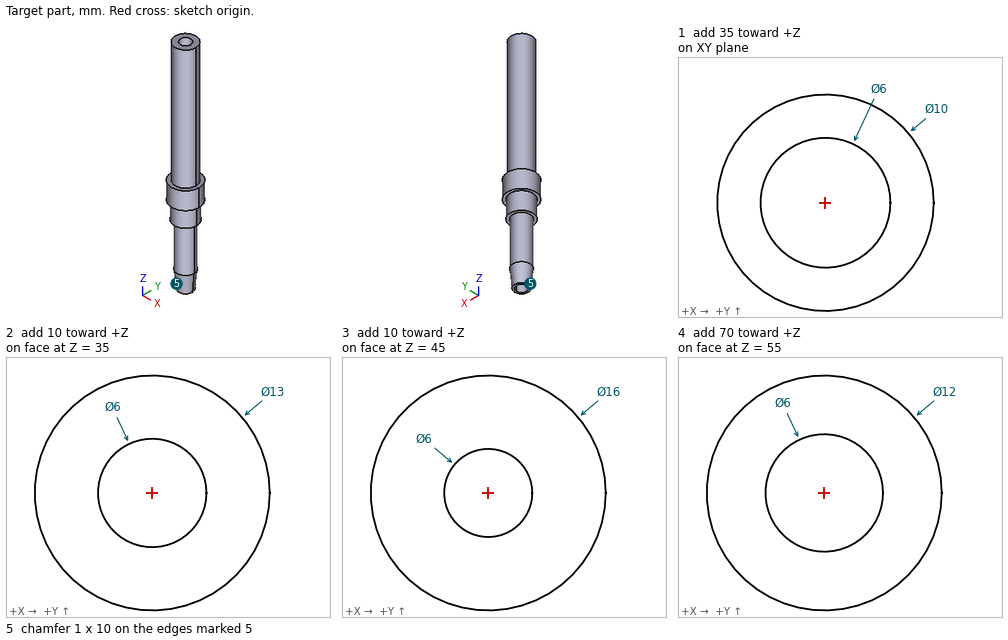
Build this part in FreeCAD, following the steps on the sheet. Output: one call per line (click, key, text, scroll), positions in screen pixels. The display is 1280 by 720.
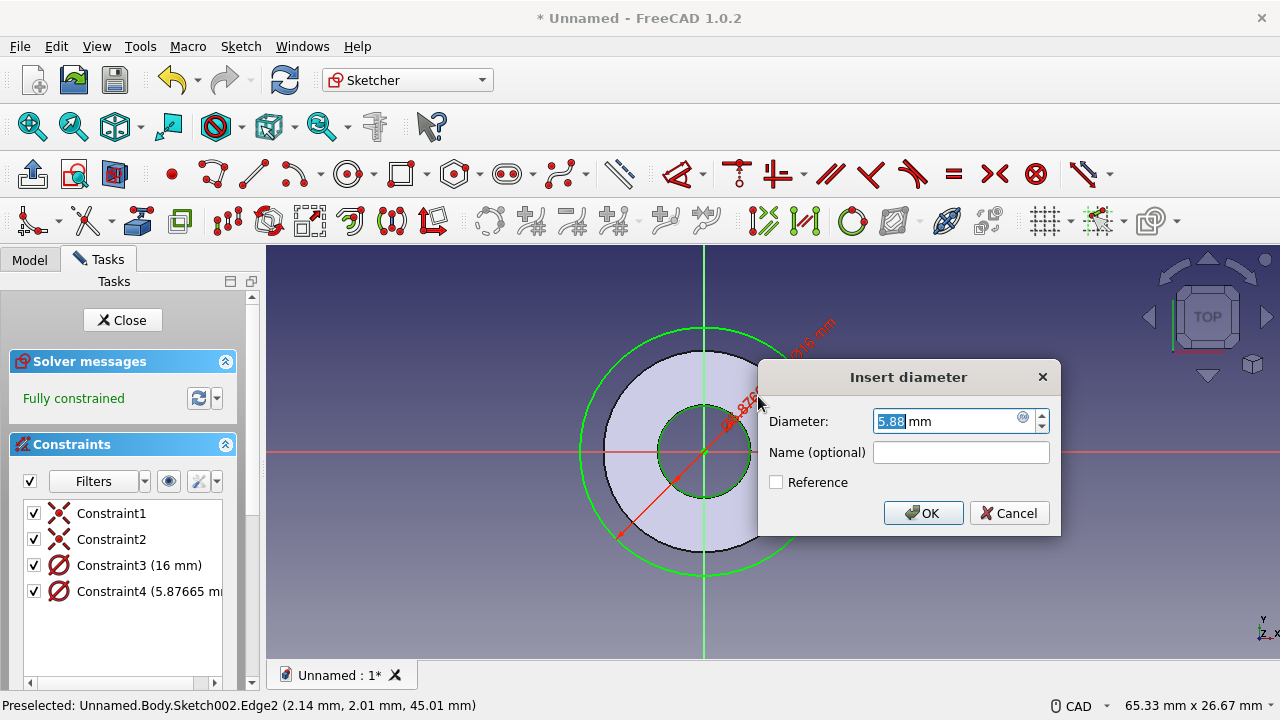
text(6)
key(Return)
key(Escape)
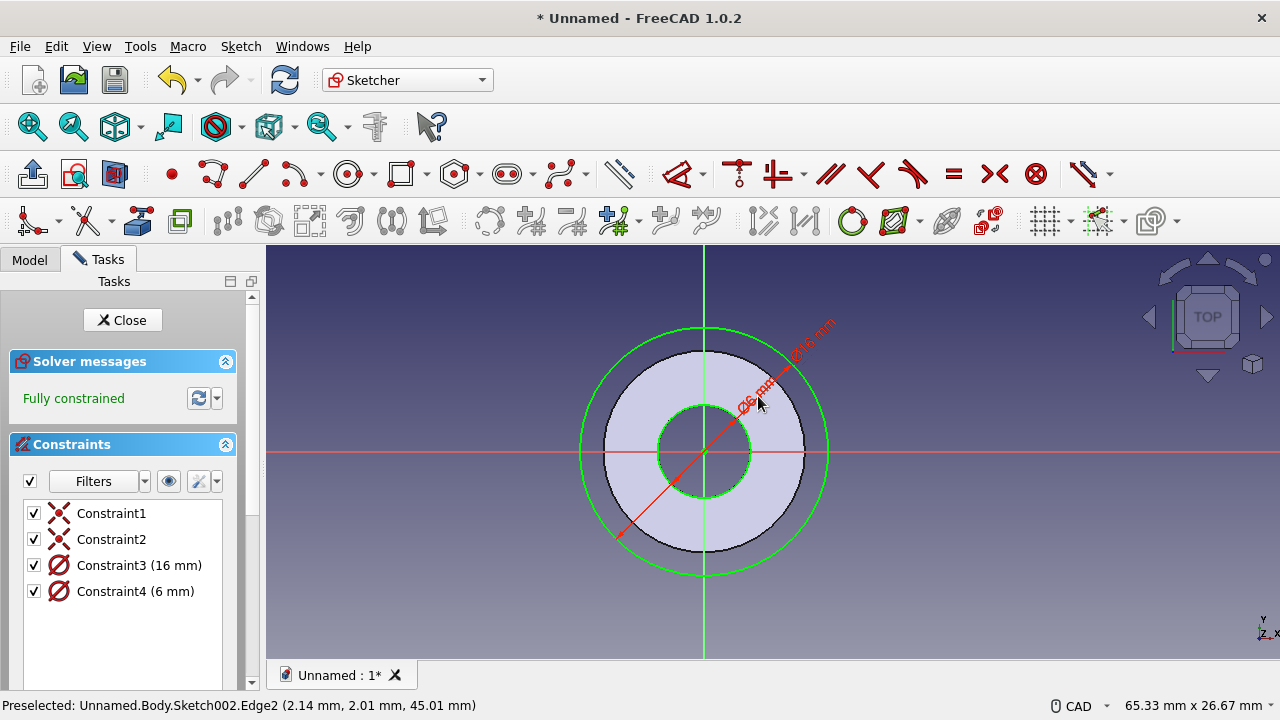
click(123, 320)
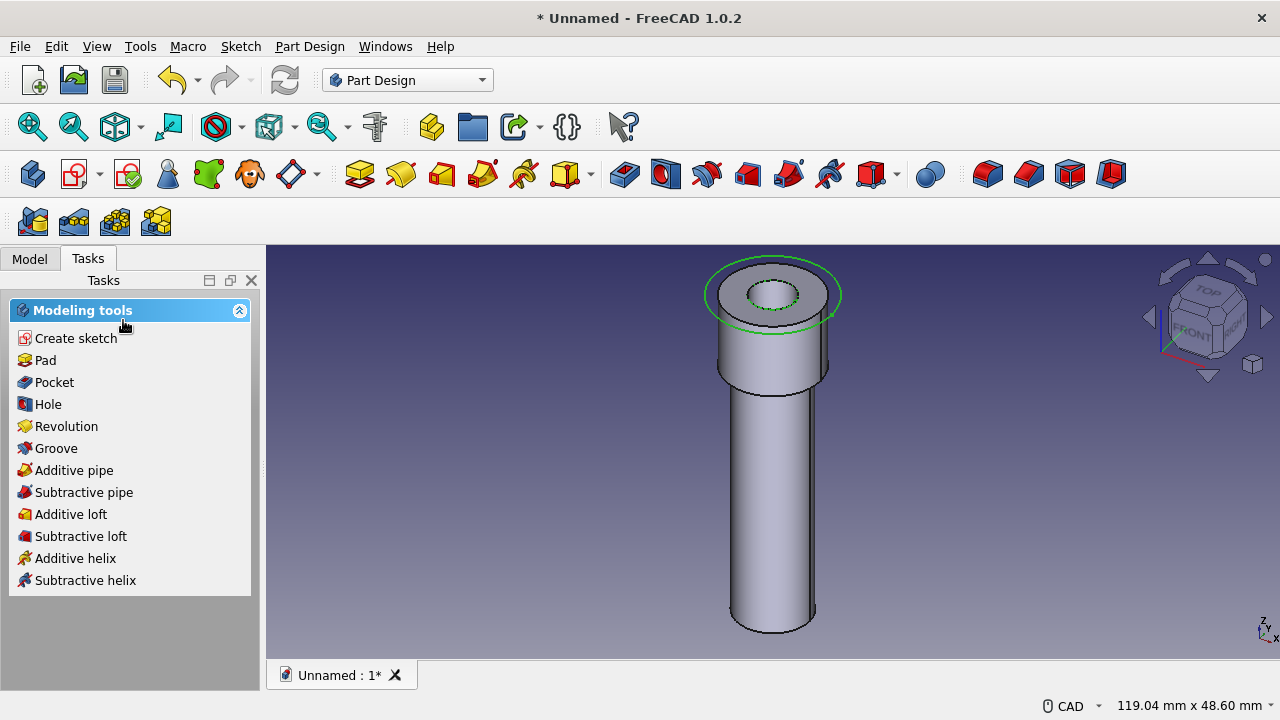
click(360, 174)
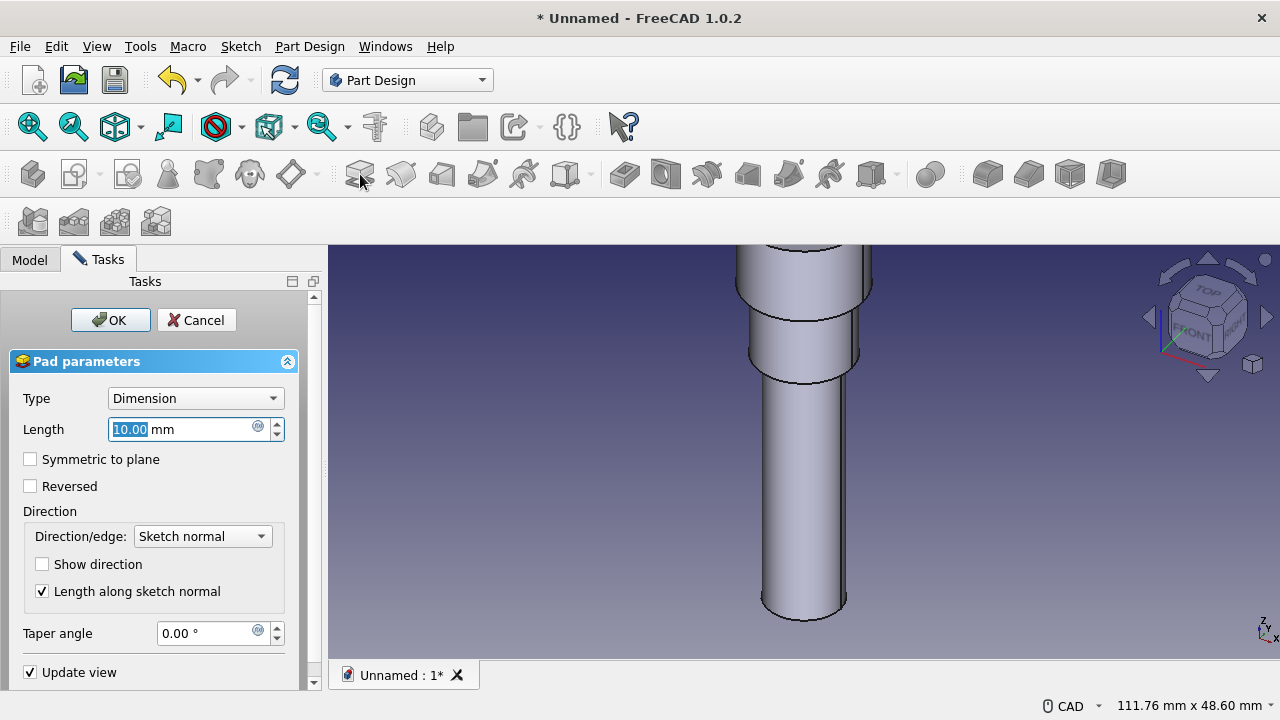
text(10)
key(Tab)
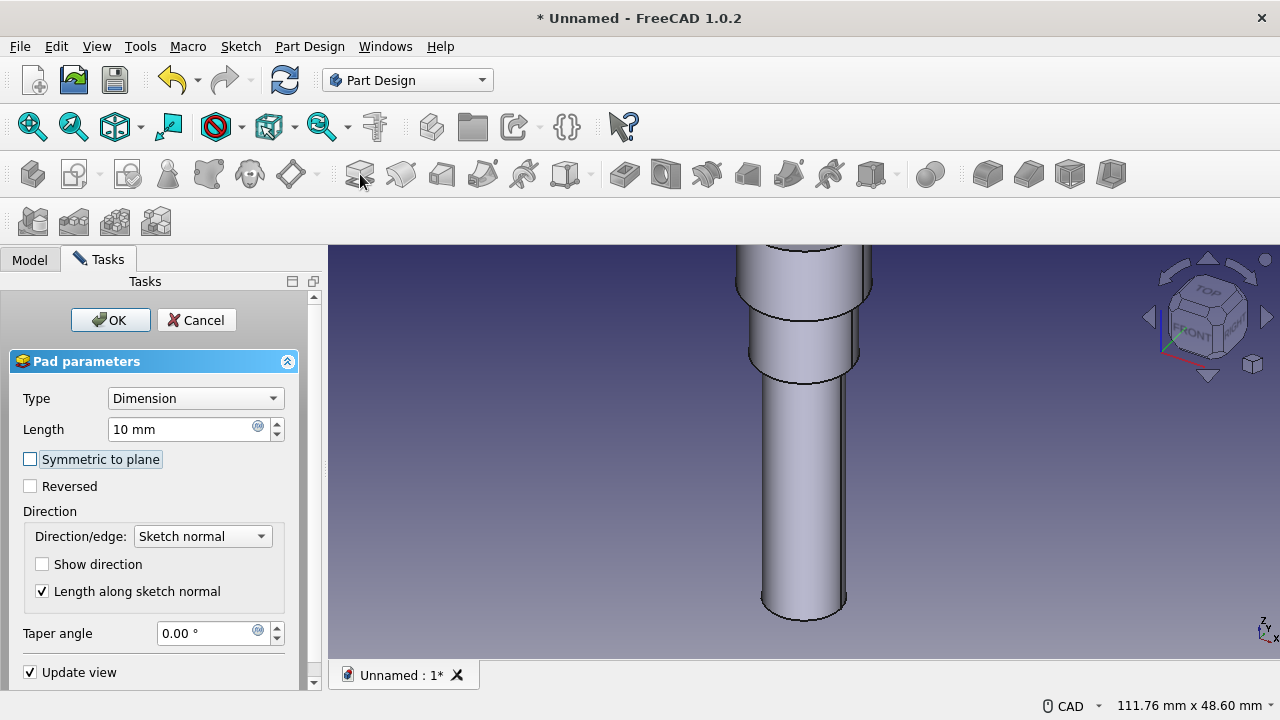
click(111, 320)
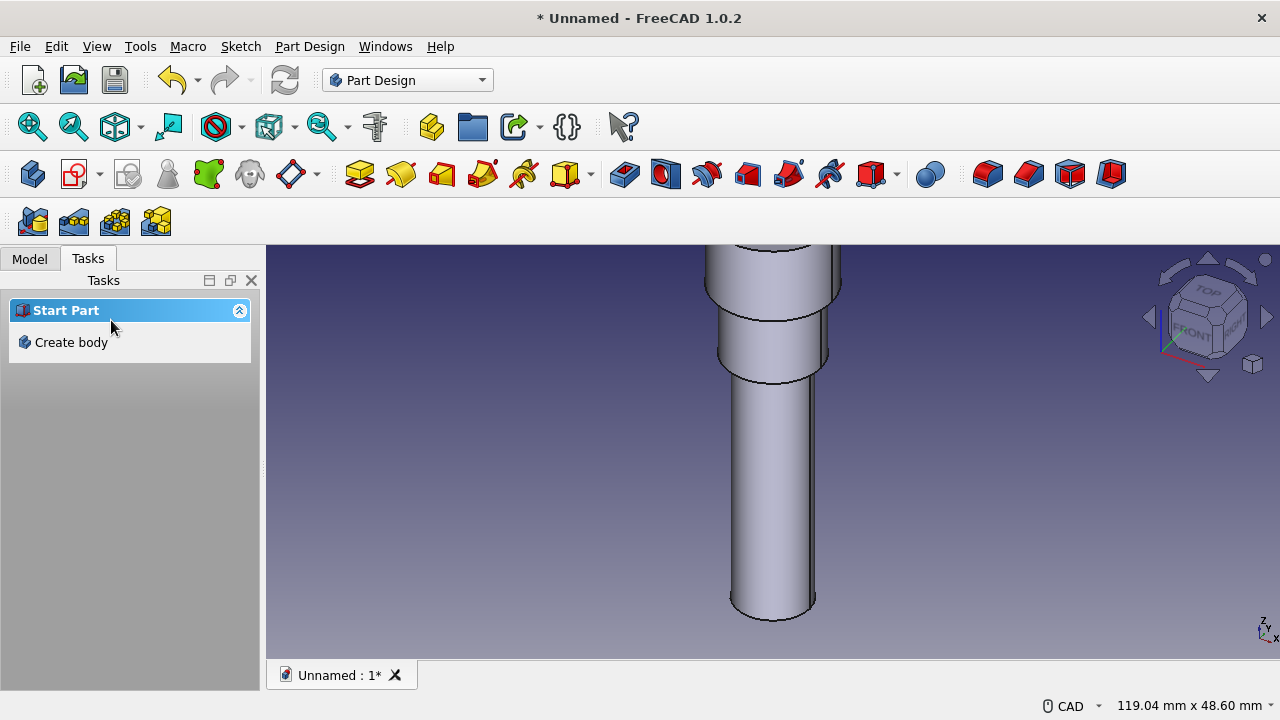
click(33, 128)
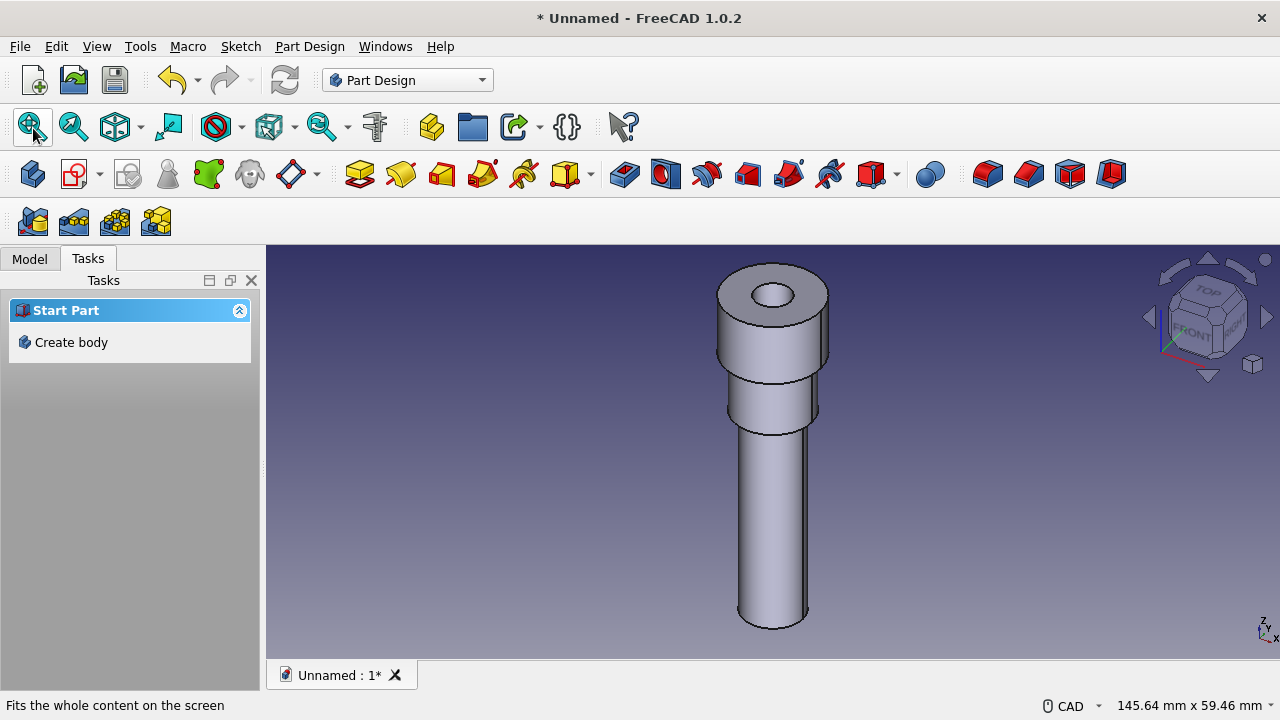
click(803, 283)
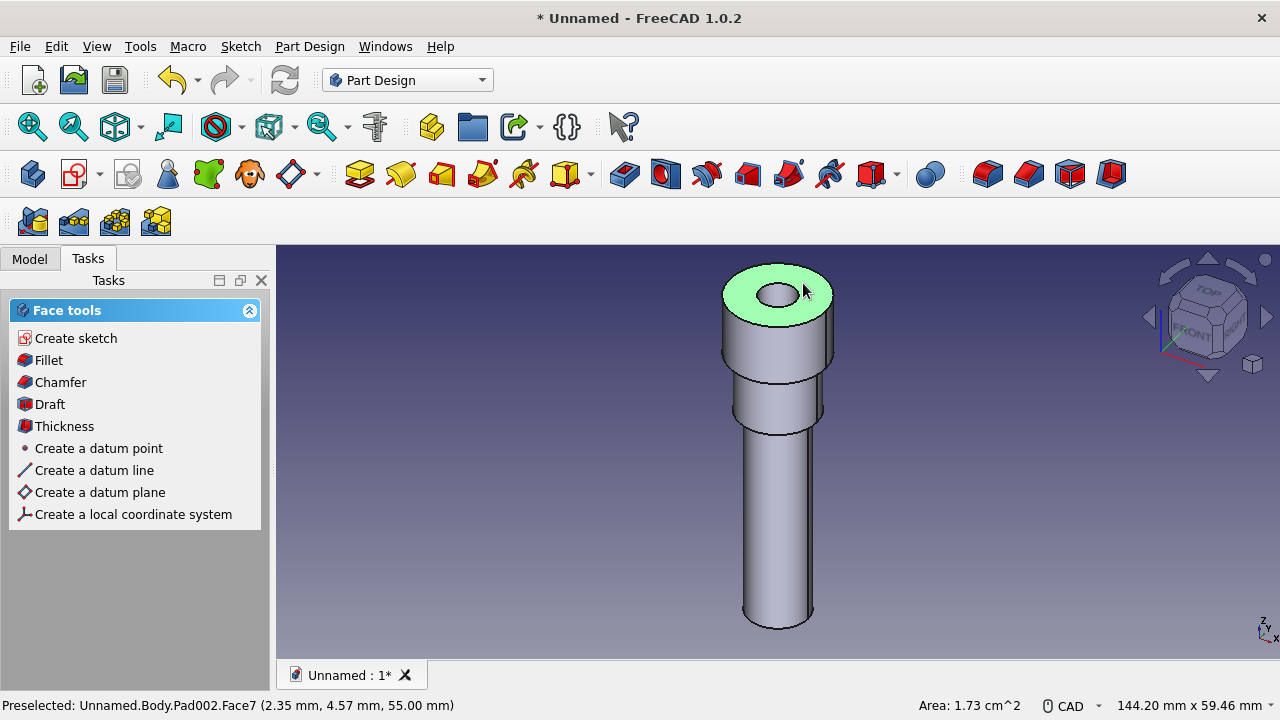
click(74, 174)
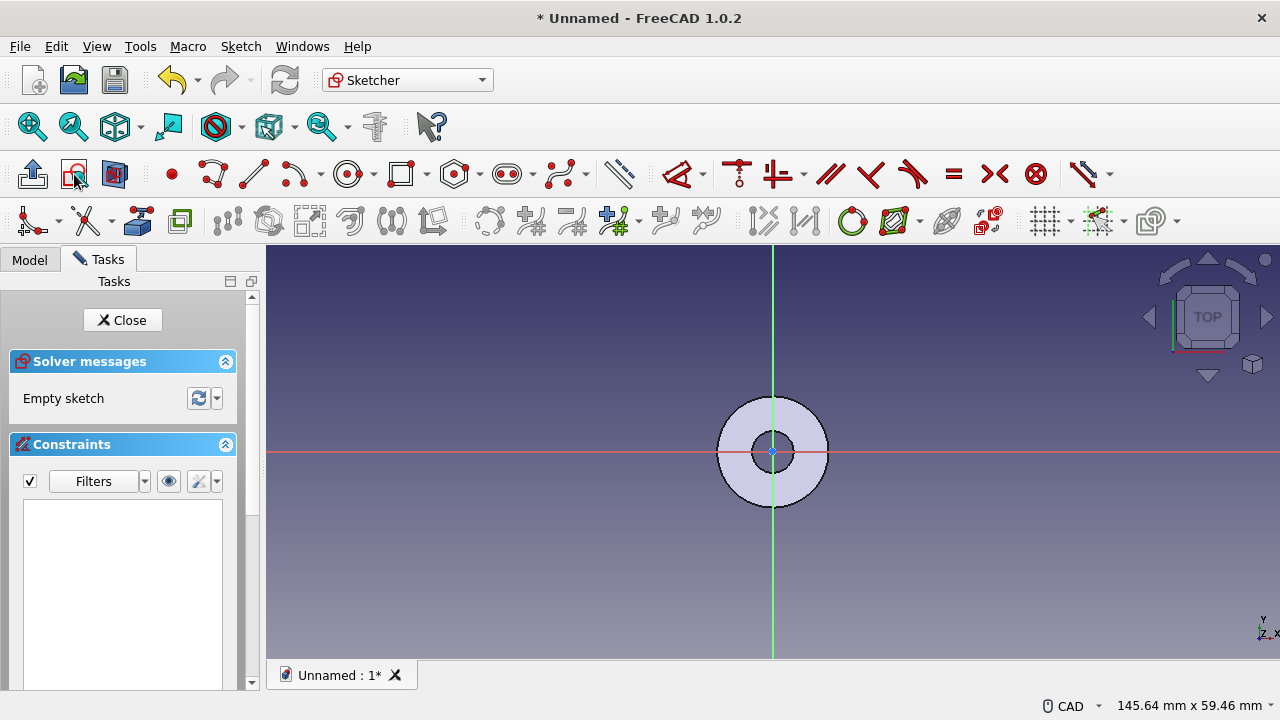
scroll(802, 452, up, 6)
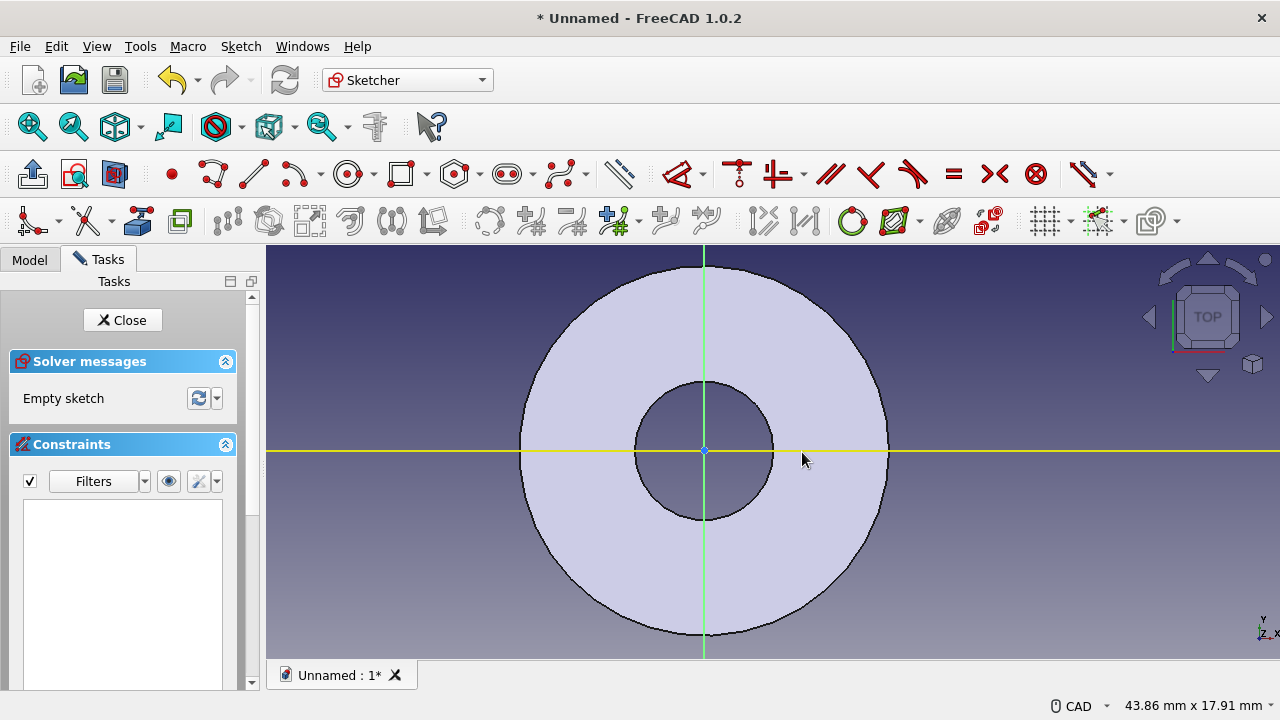
click(348, 174)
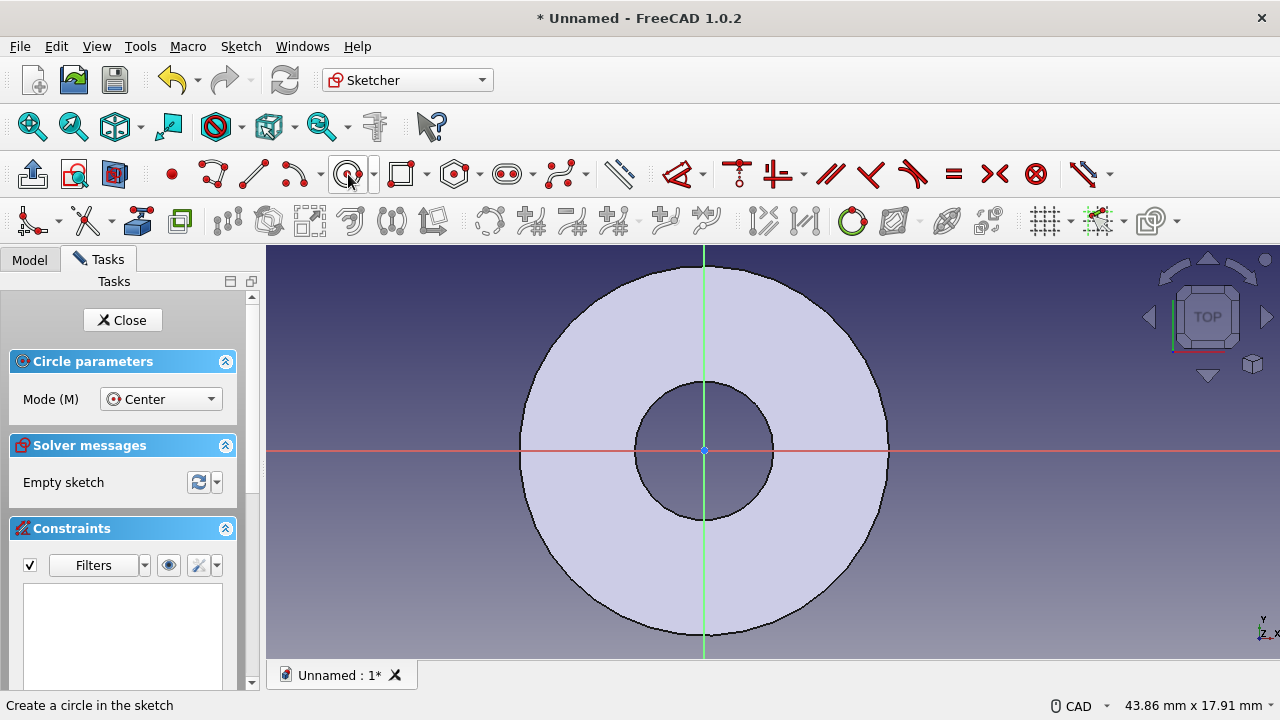
click(704, 451)
click(802, 353)